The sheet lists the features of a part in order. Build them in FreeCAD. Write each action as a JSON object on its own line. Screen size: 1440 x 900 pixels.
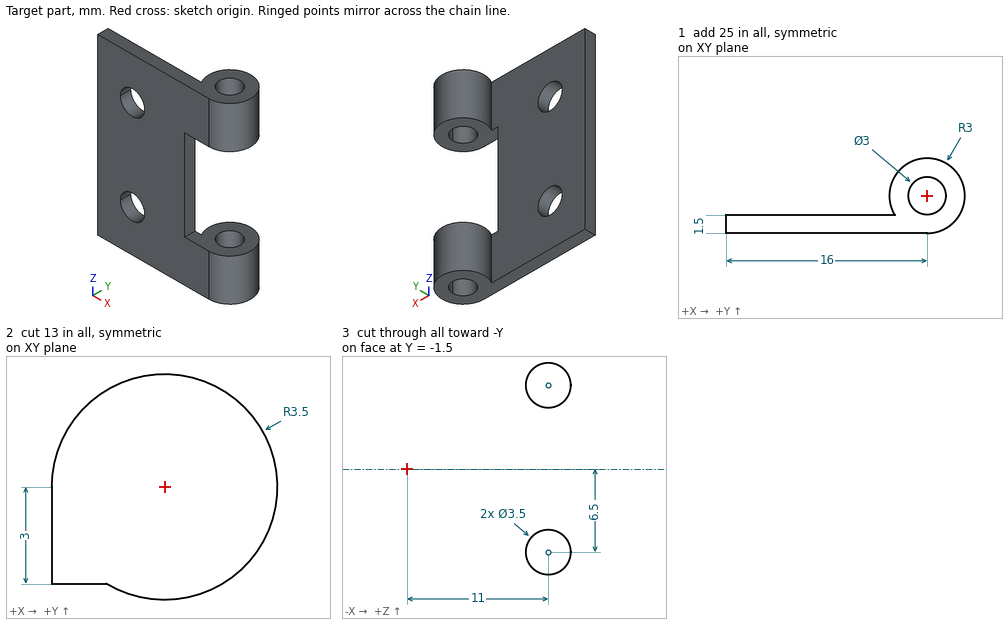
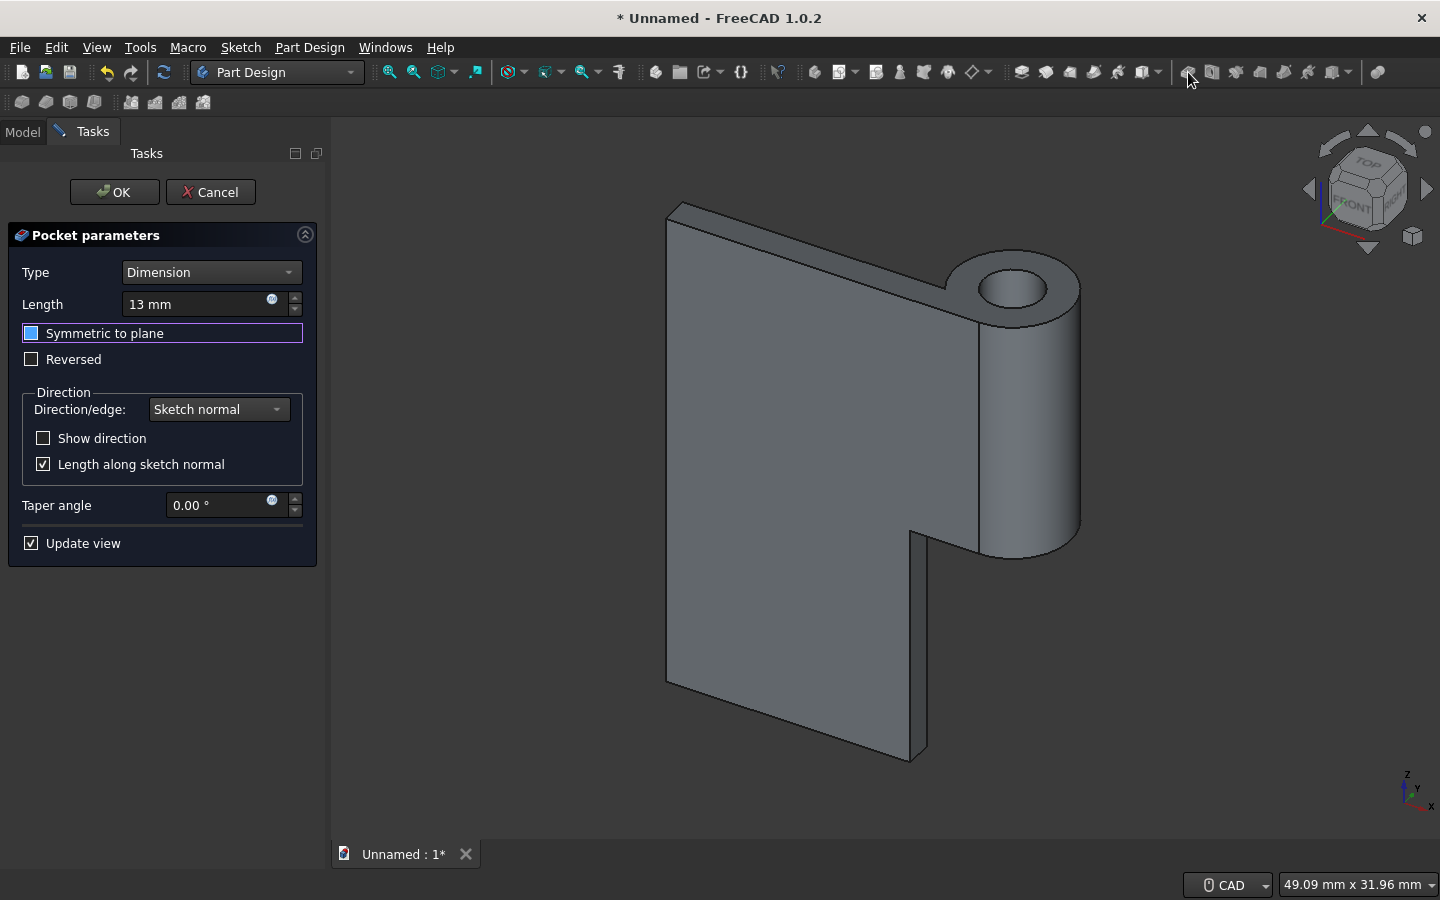
{"action": "left_click", "coordinate": [30, 333]}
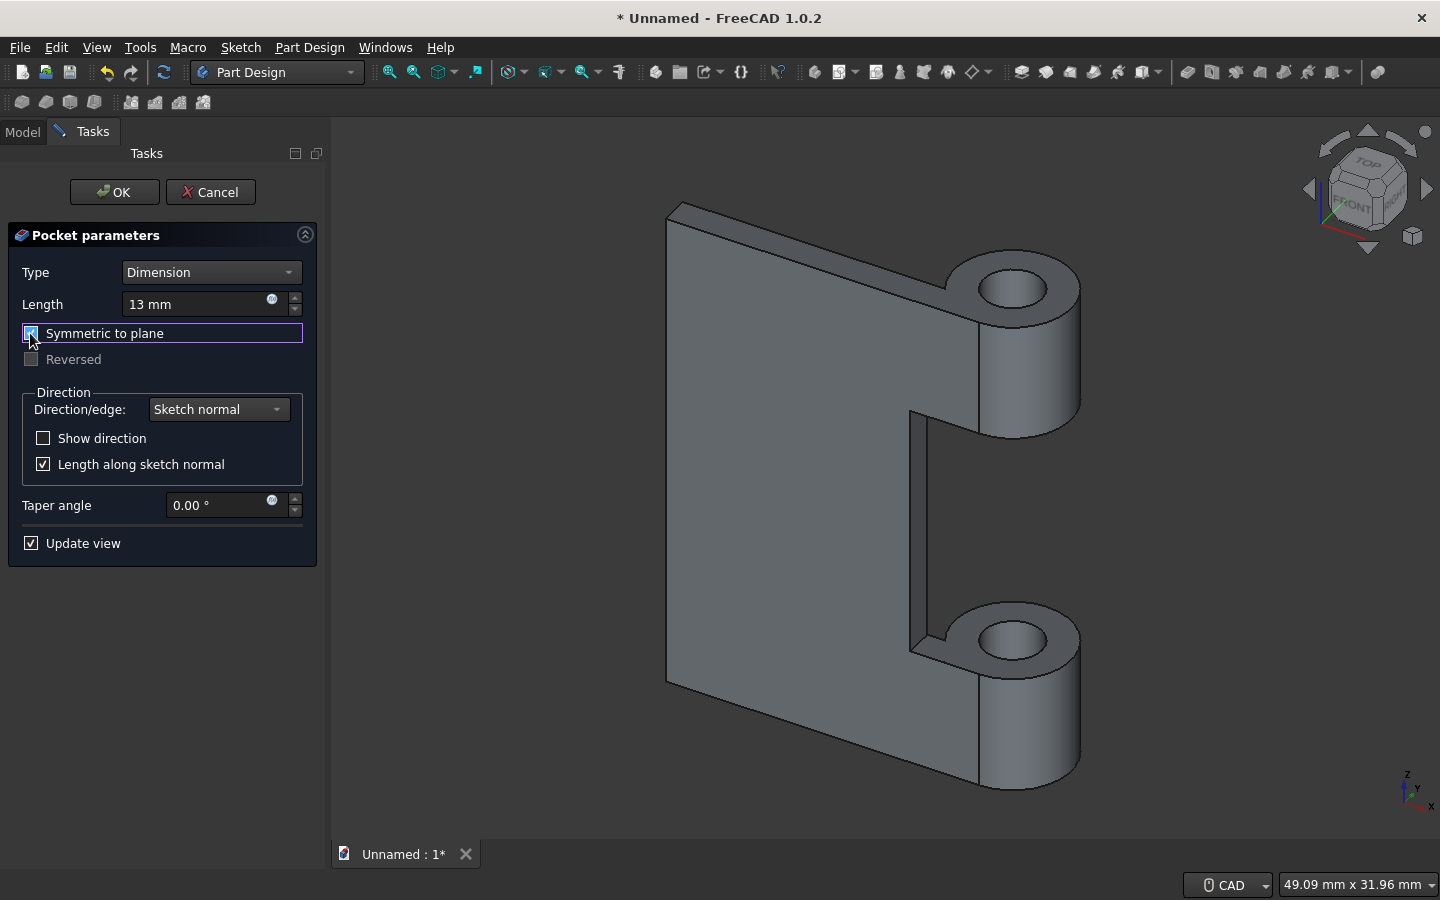
{"action": "left_click", "coordinate": [115, 192]}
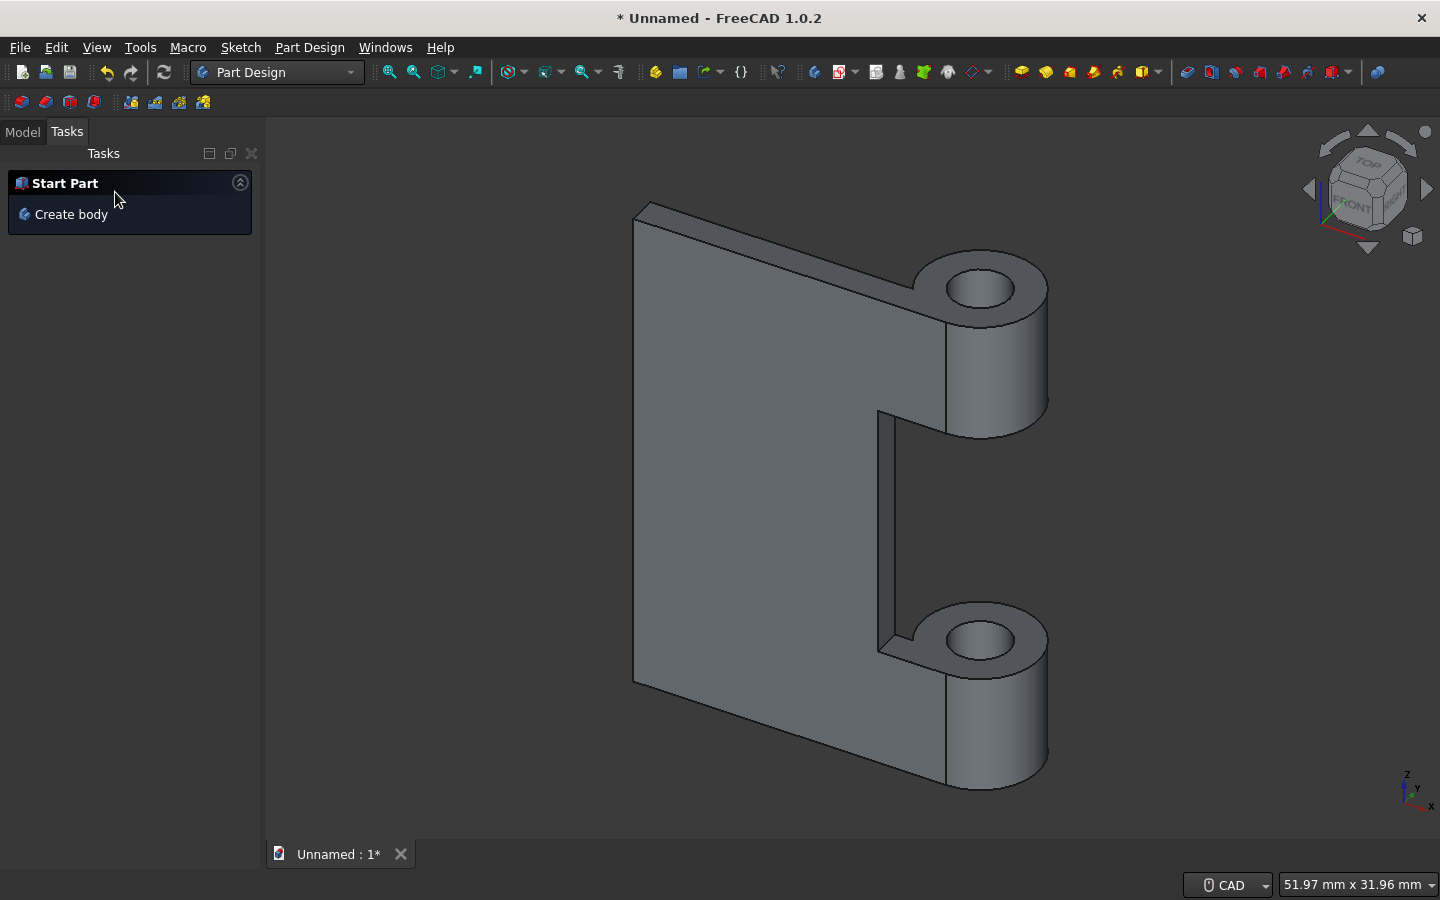
{"action": "key", "text": "4"}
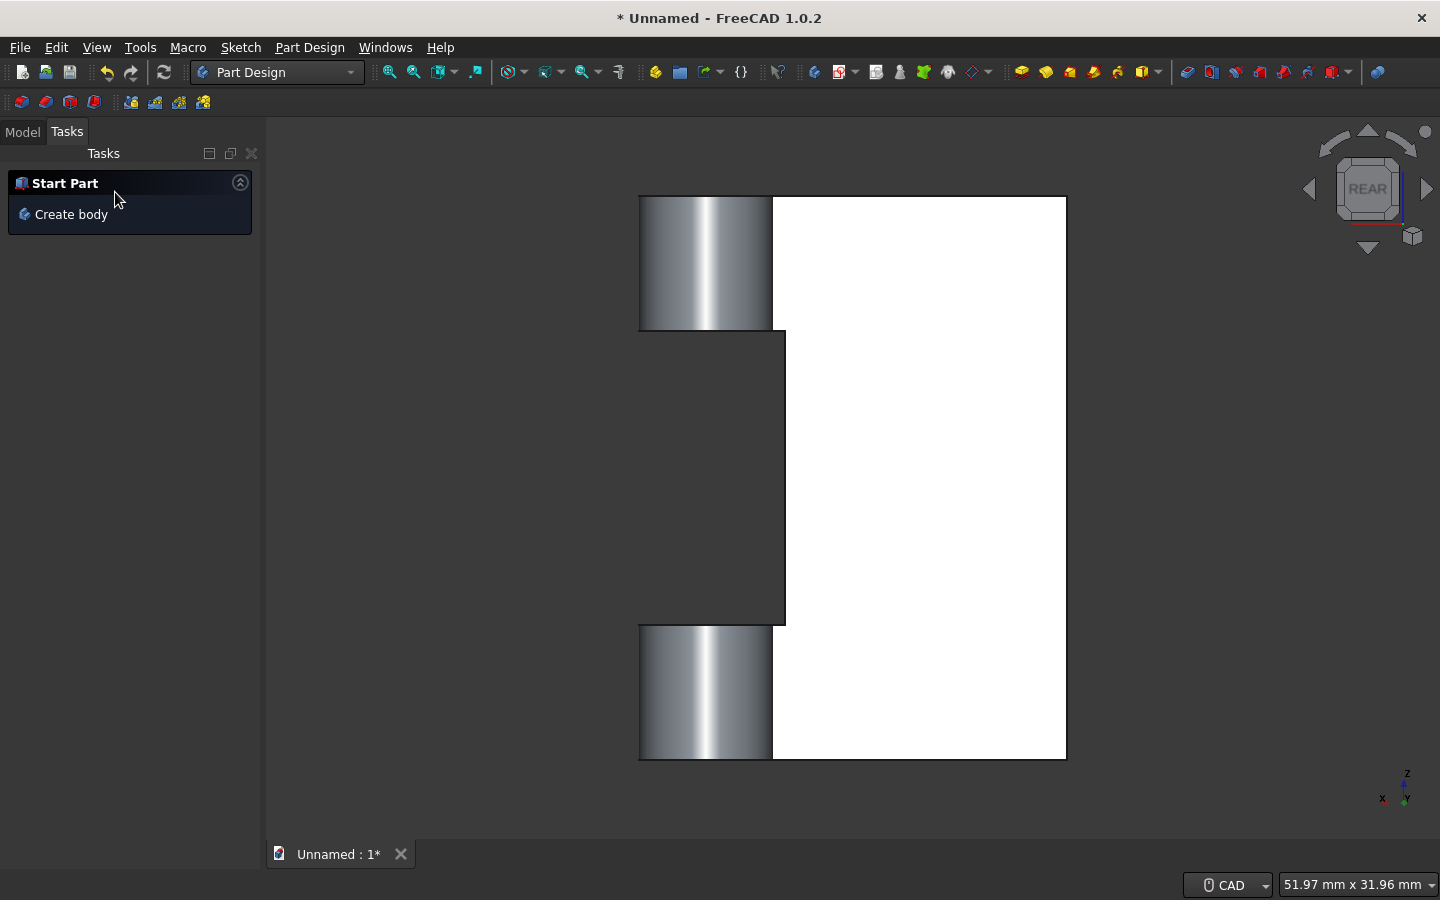
{"action": "left_click", "coordinate": [916, 396]}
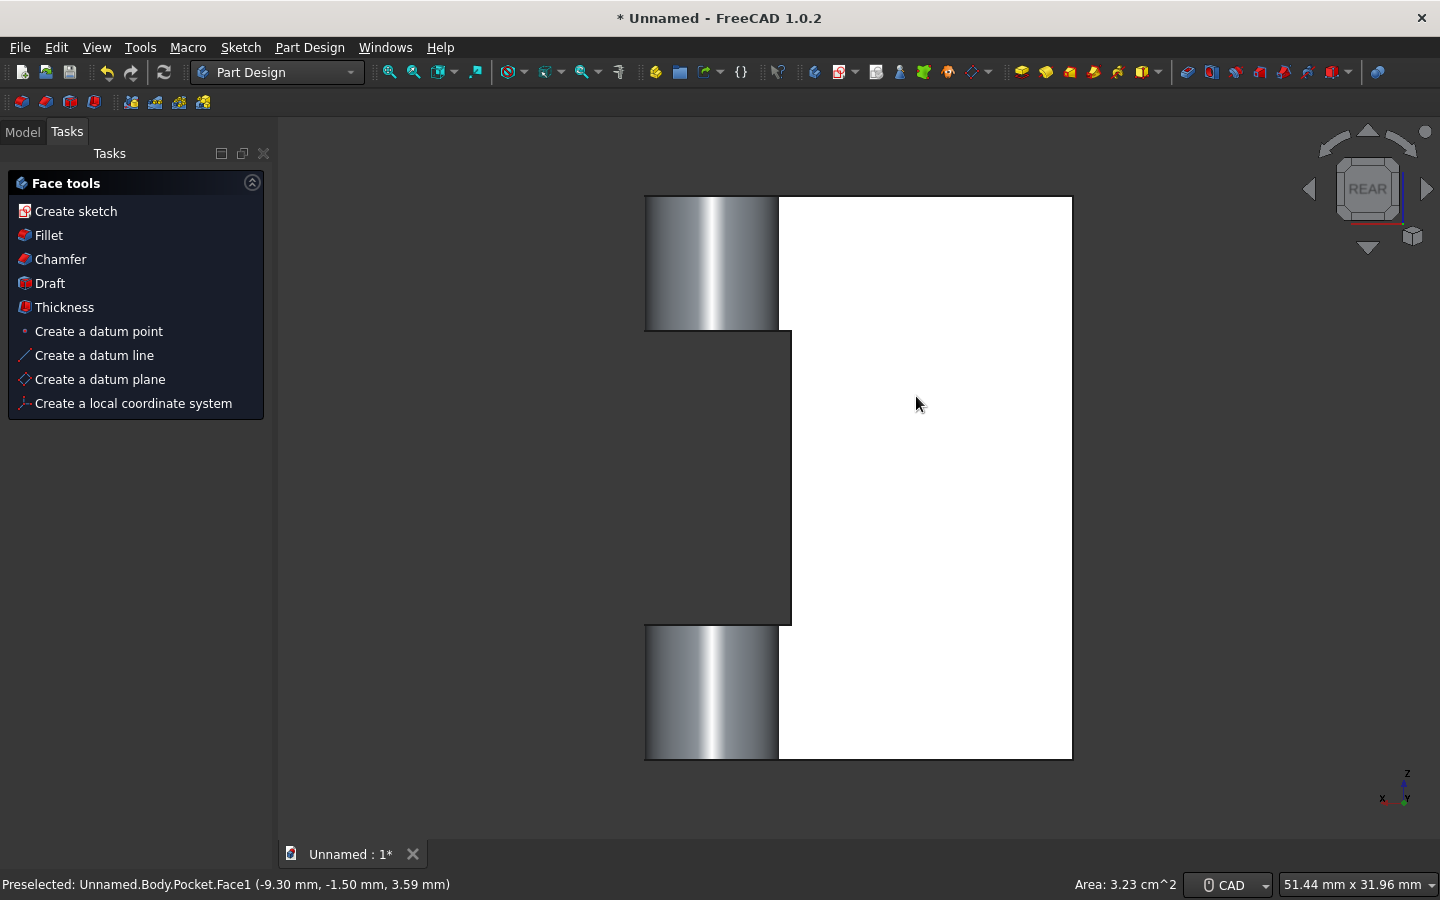
{"action": "left_click", "coordinate": [840, 72]}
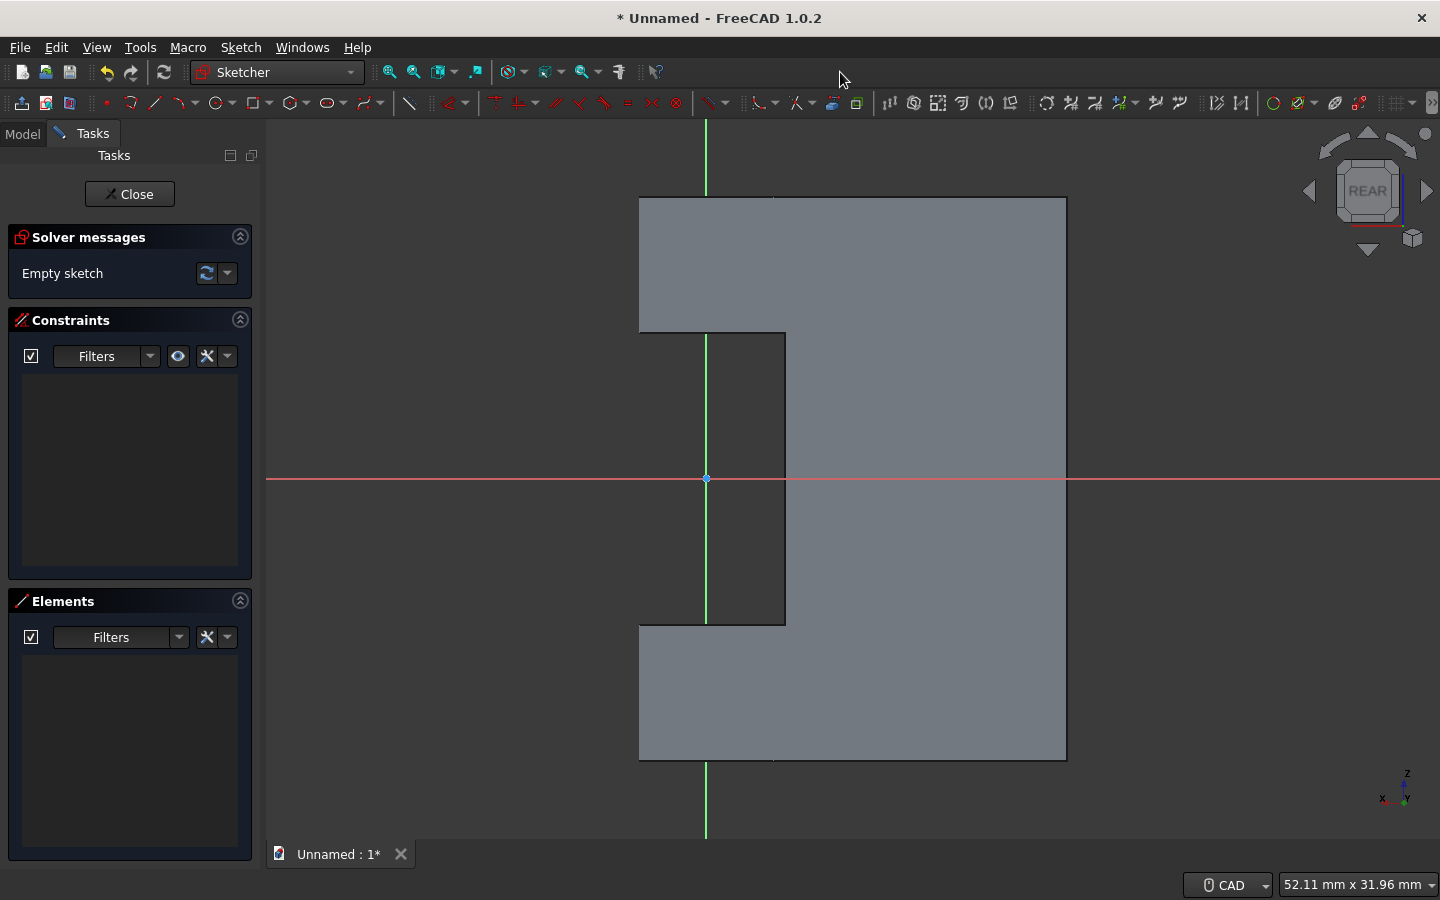
{"action": "left_click", "coordinate": [216, 104]}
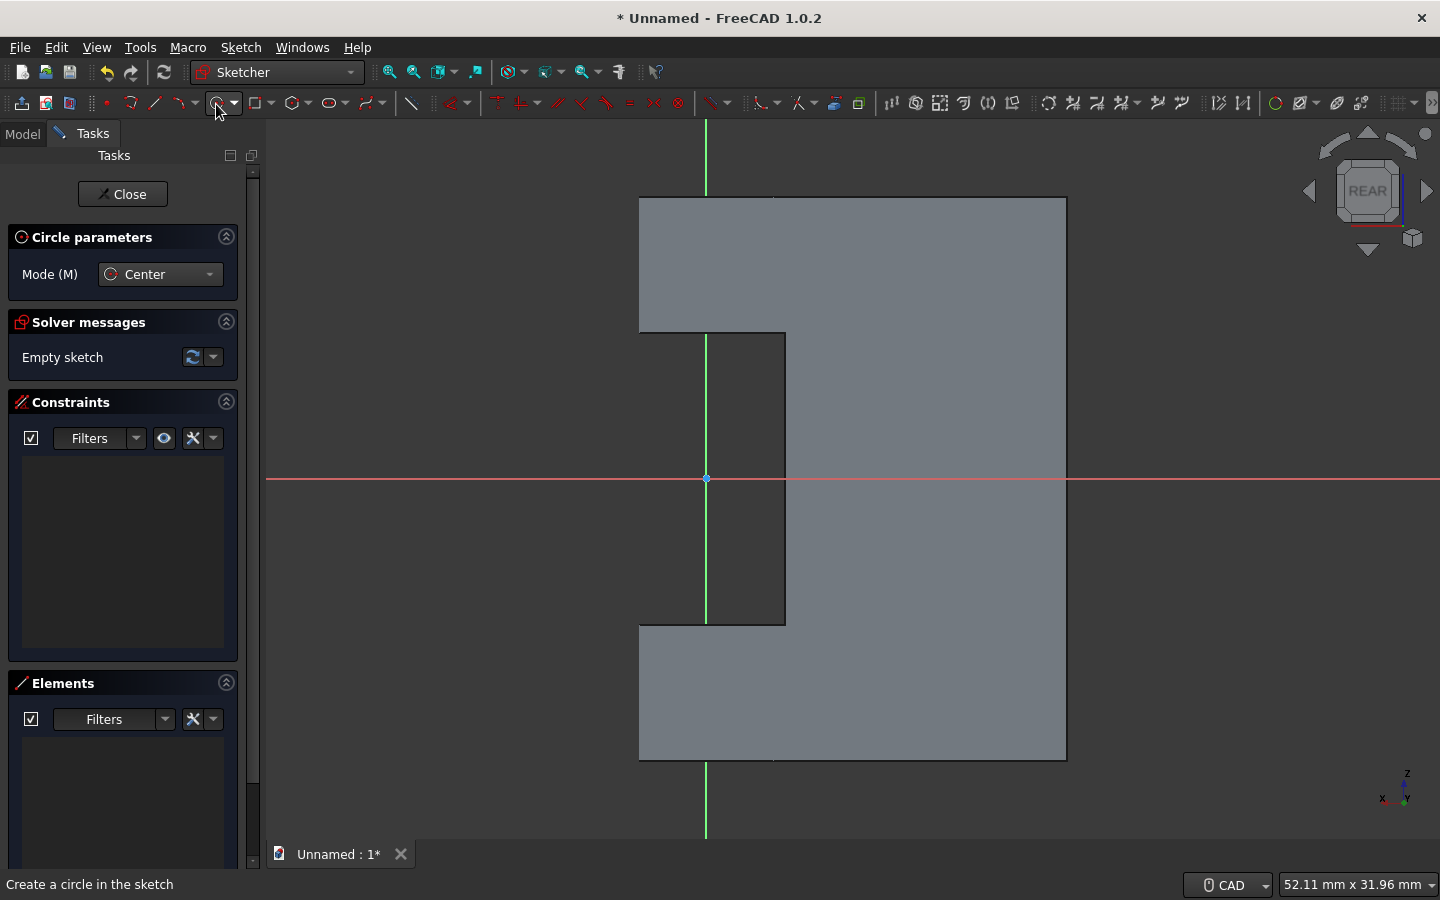
{"action": "left_click", "coordinate": [954, 625]}
{"action": "left_click", "coordinate": [982, 598]}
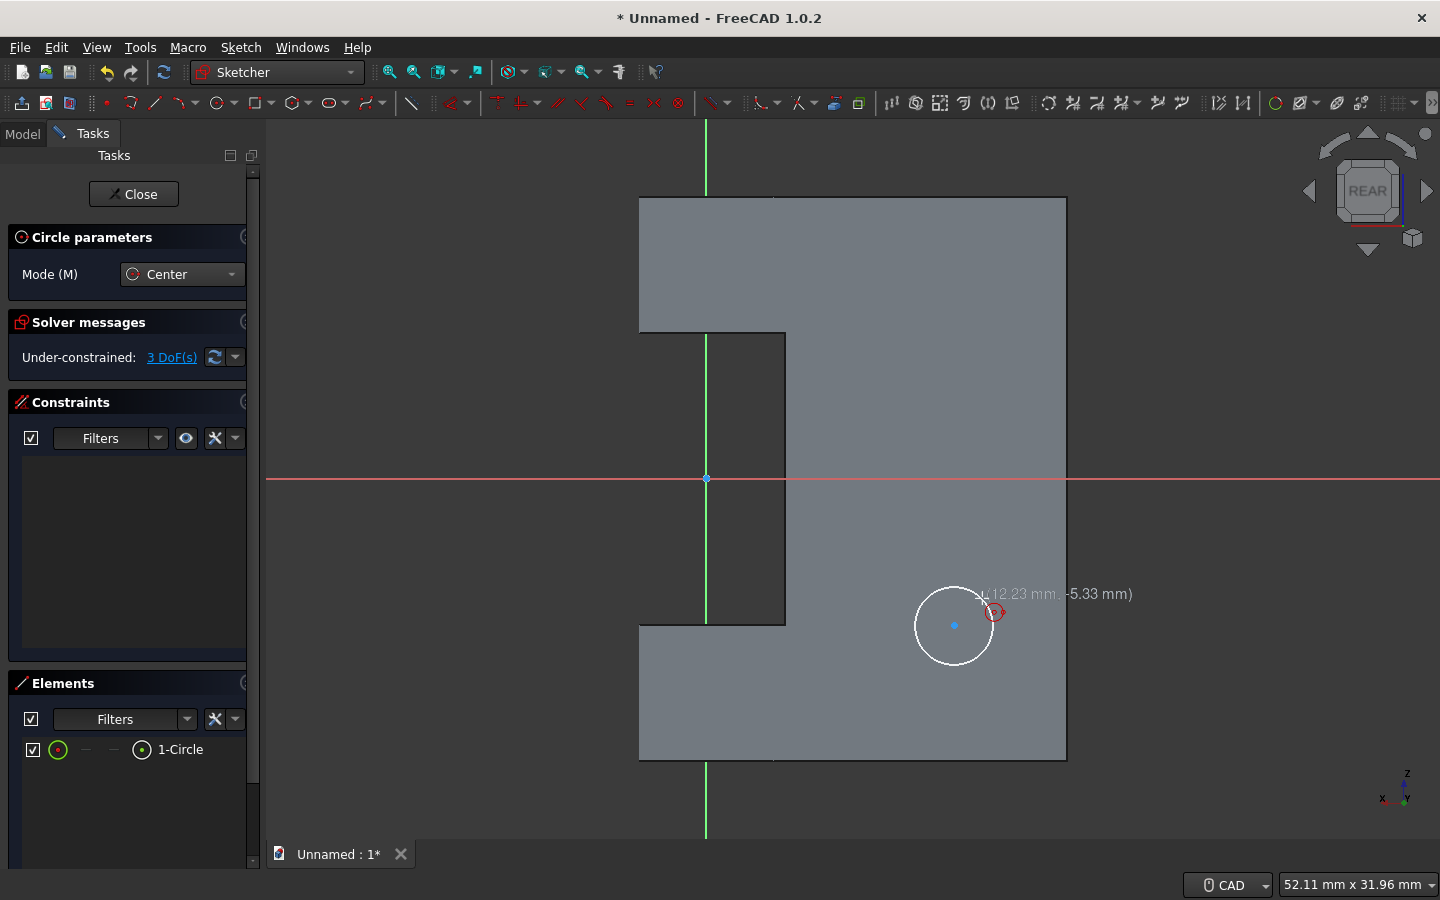
{"action": "left_click", "coordinate": [954, 333]}
{"action": "left_click", "coordinate": [982, 305]}
{"action": "key", "text": "Escape"}